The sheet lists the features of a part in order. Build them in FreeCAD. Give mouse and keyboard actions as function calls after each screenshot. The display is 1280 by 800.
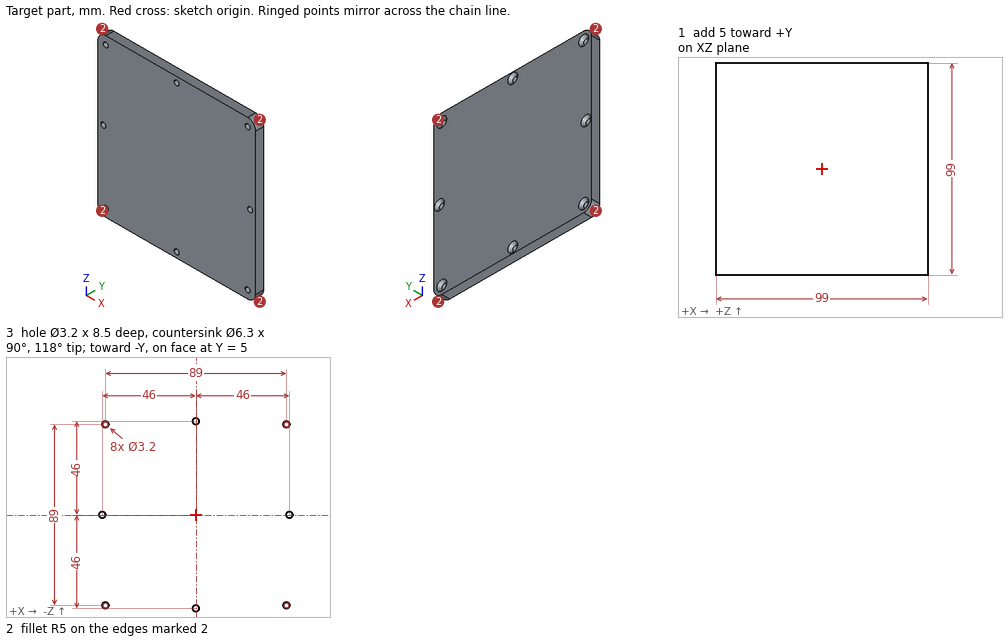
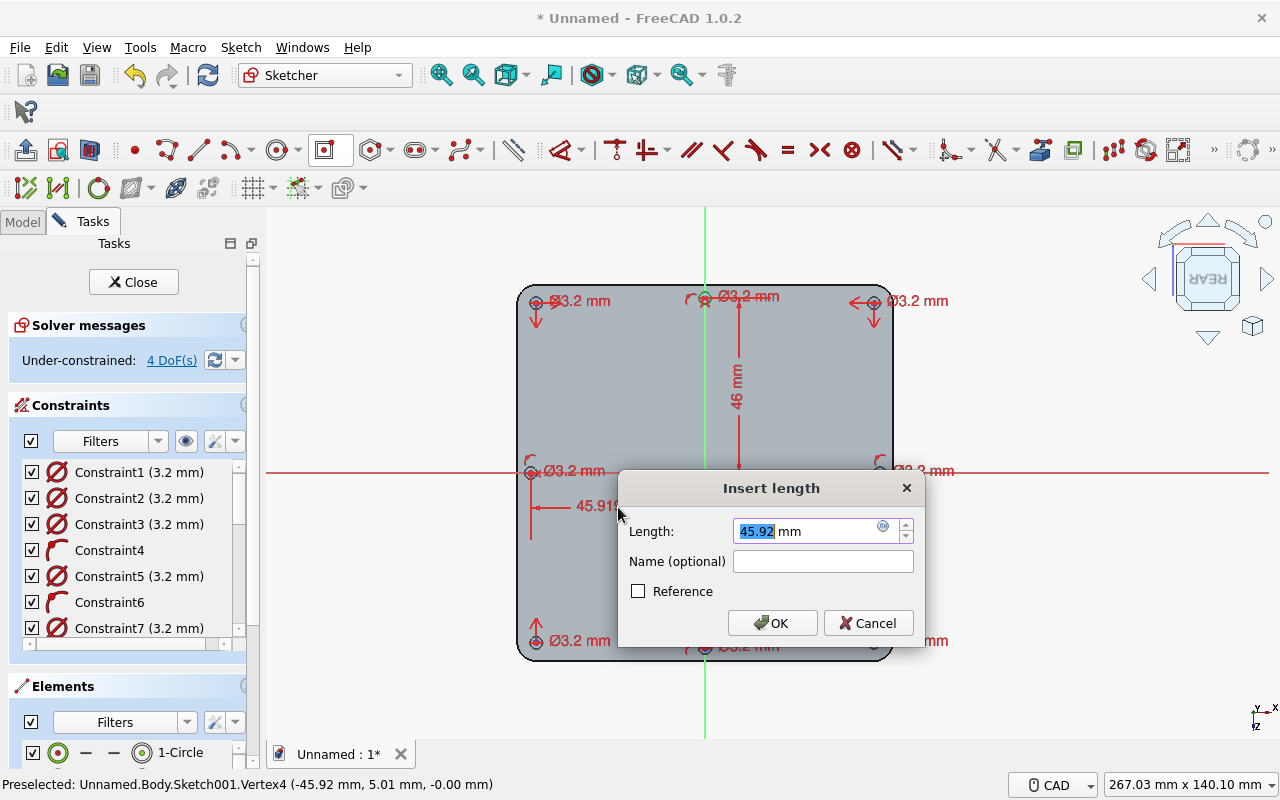
text(46)
key(Return)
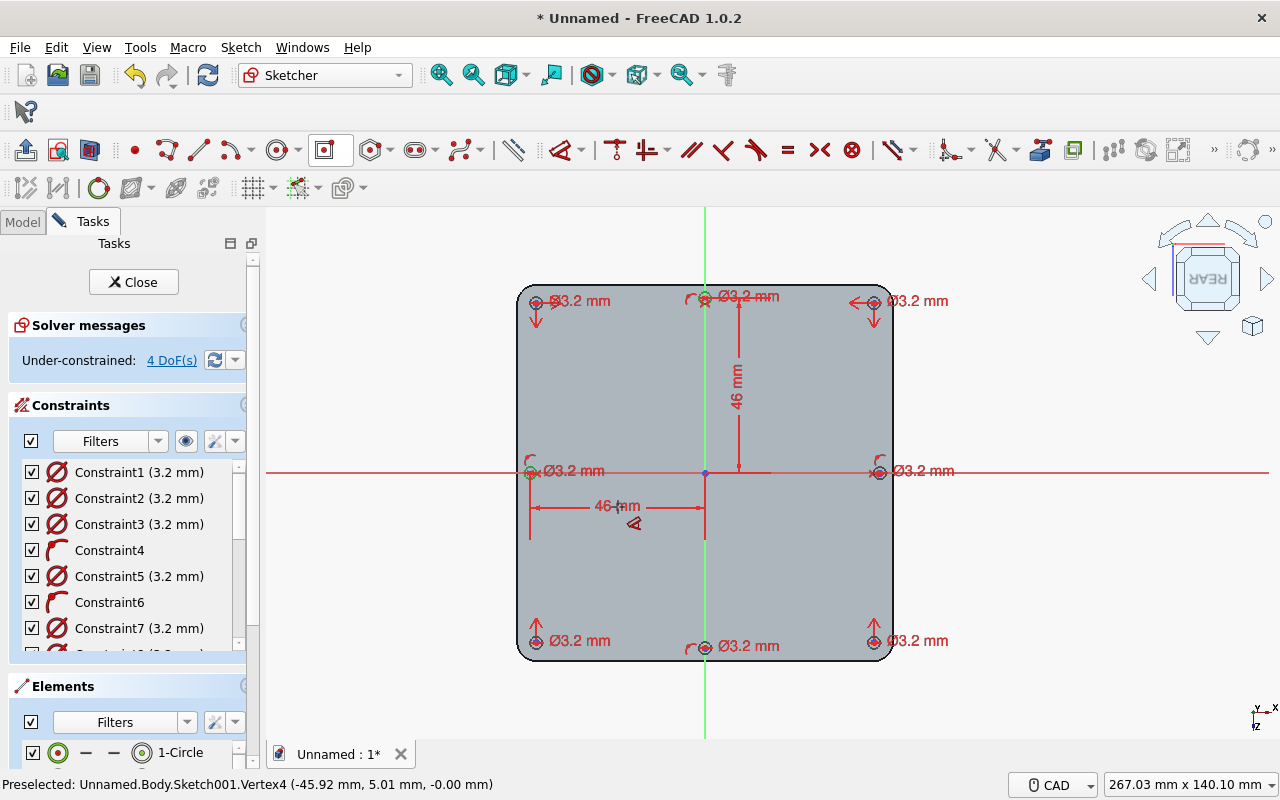
click(705, 648)
click(739, 561)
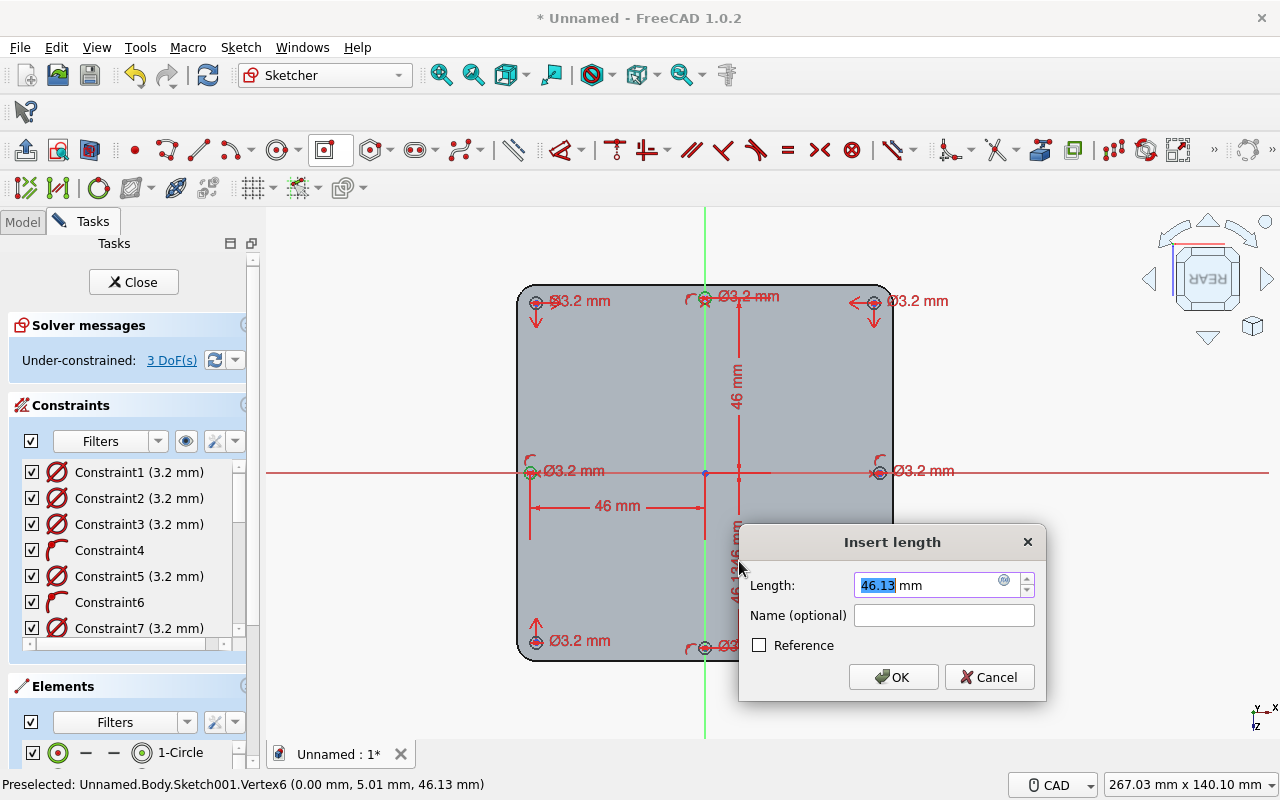
text(46)
key(Return)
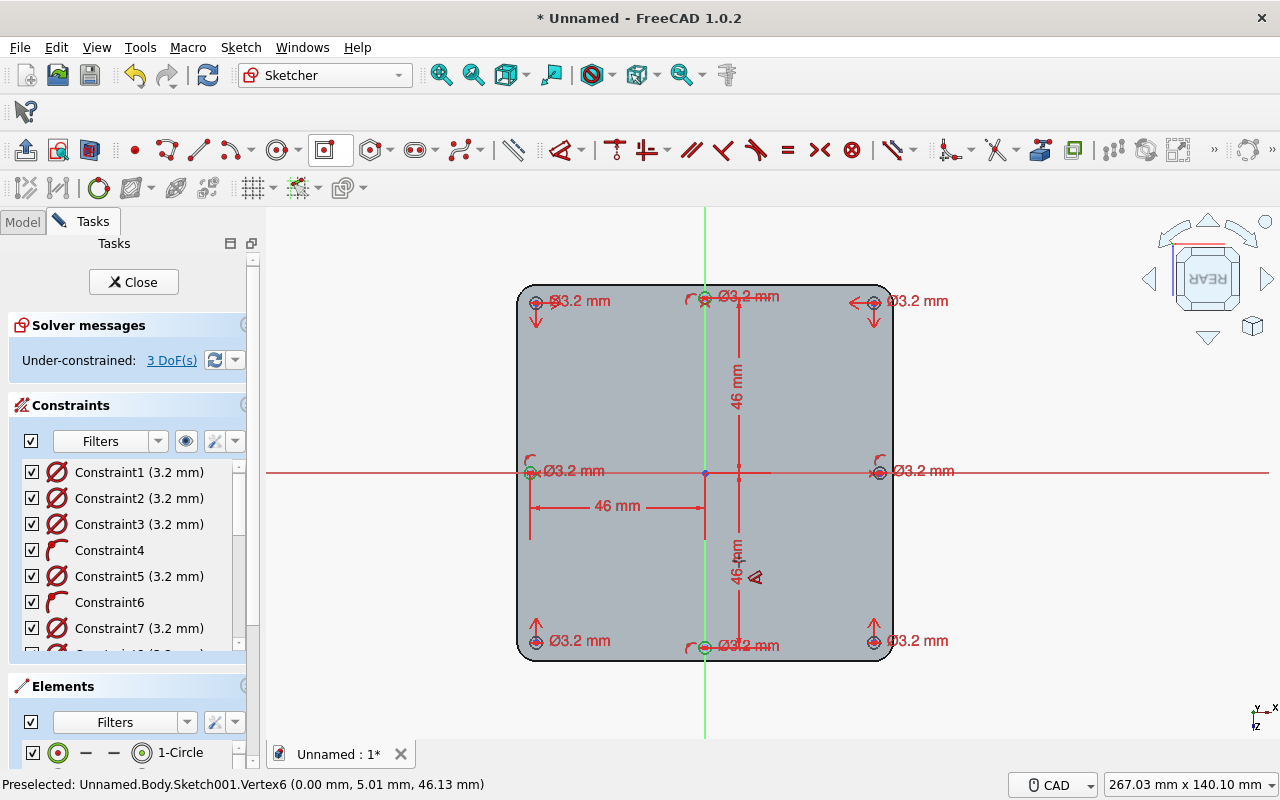
click(880, 473)
click(793, 507)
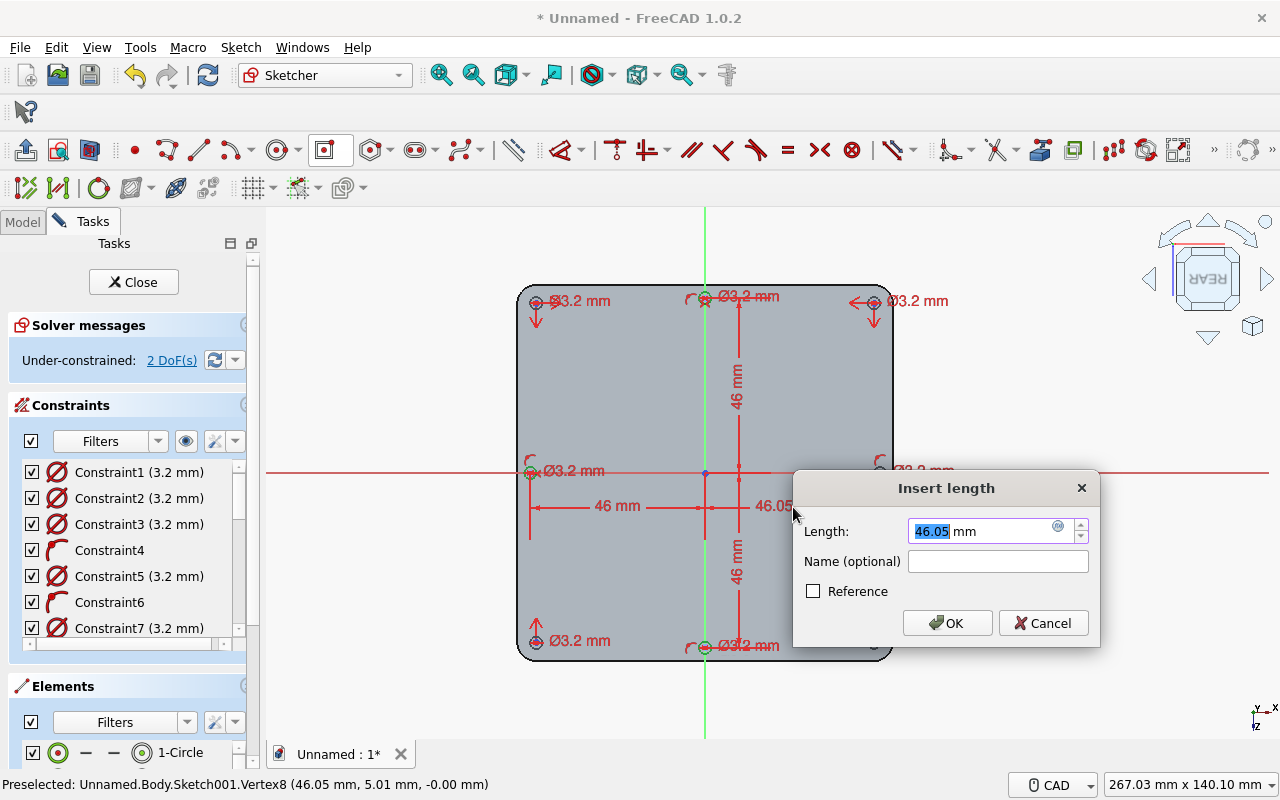
text(46)
key(Return)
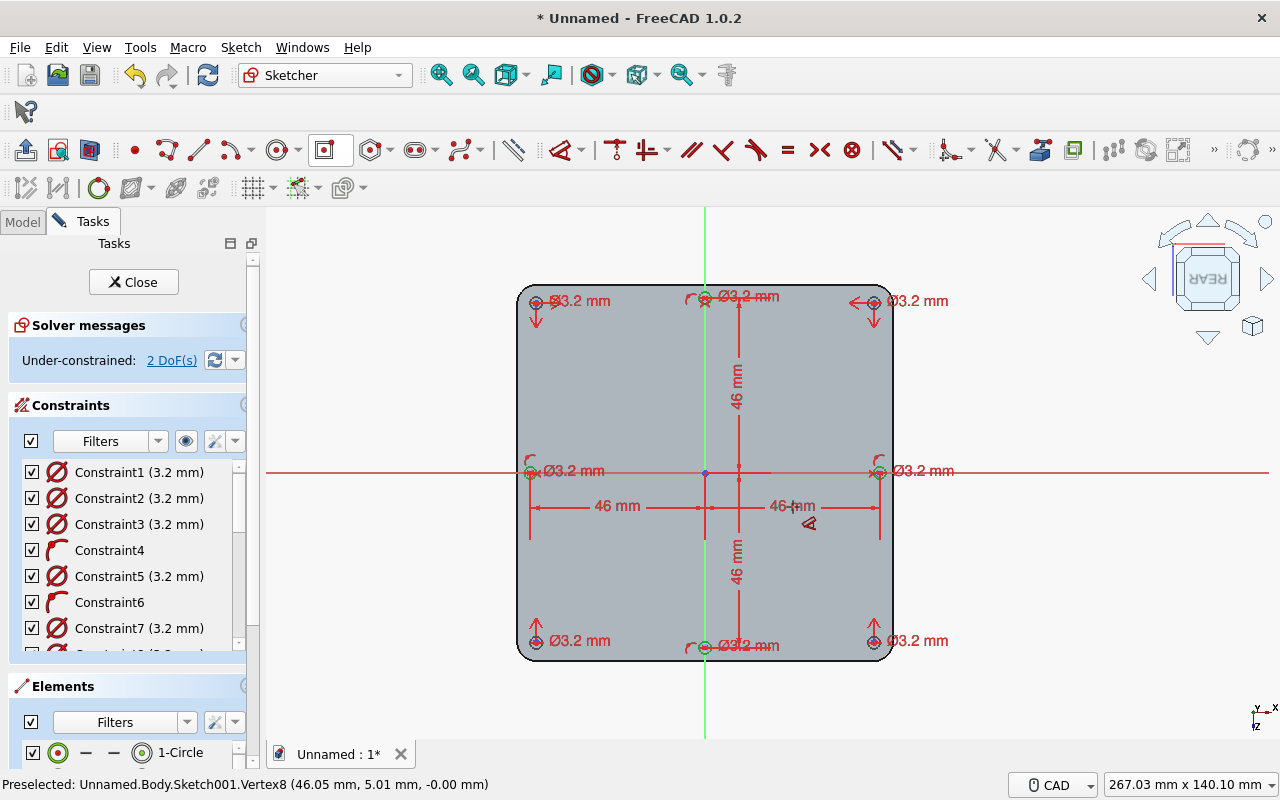
click(536, 303)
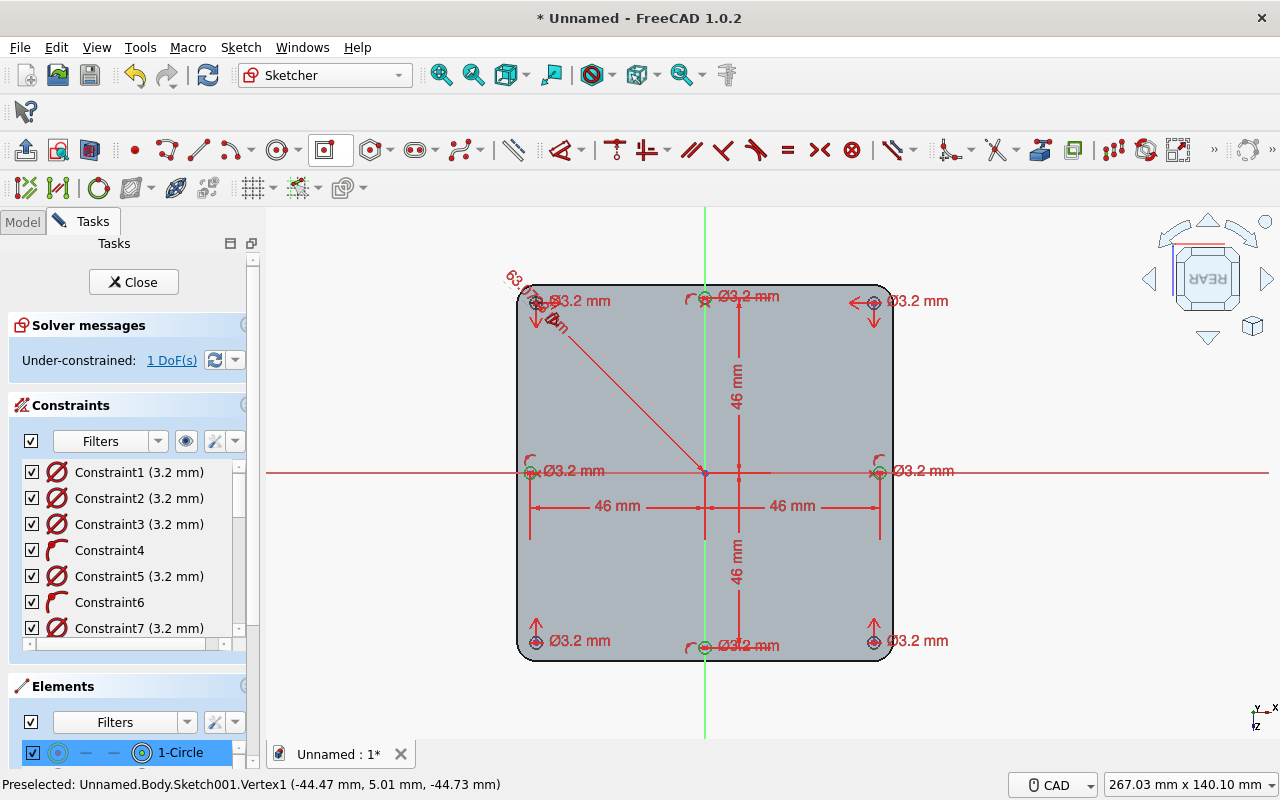
click(874, 303)
click(627, 269)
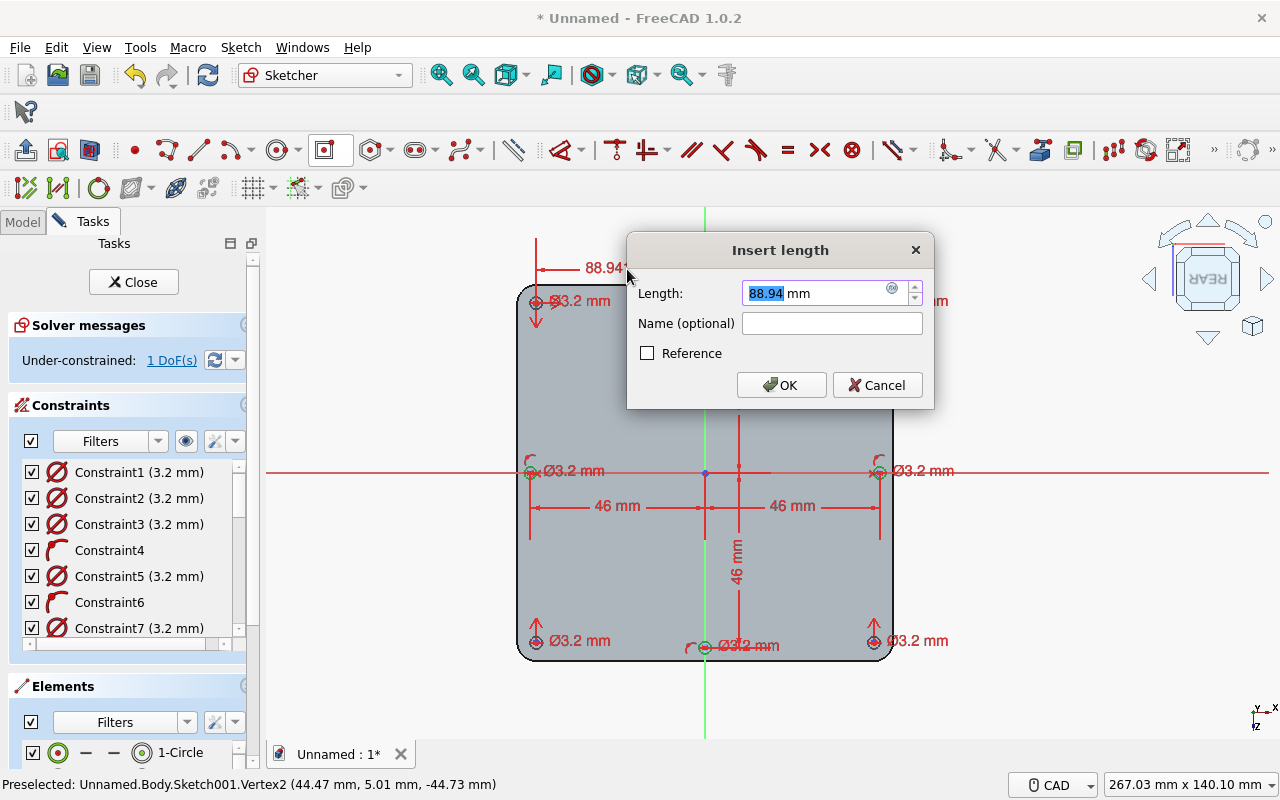
text(89)
key(Return)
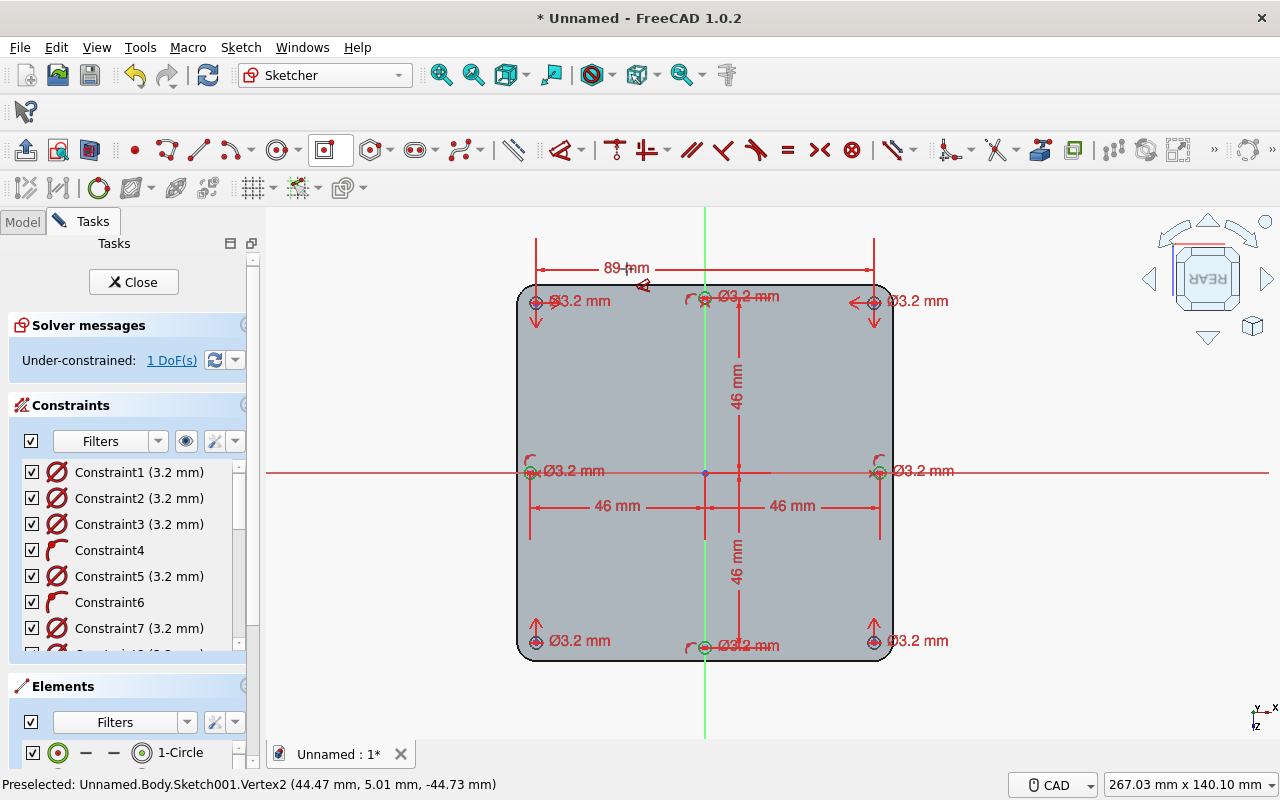
click(536, 303)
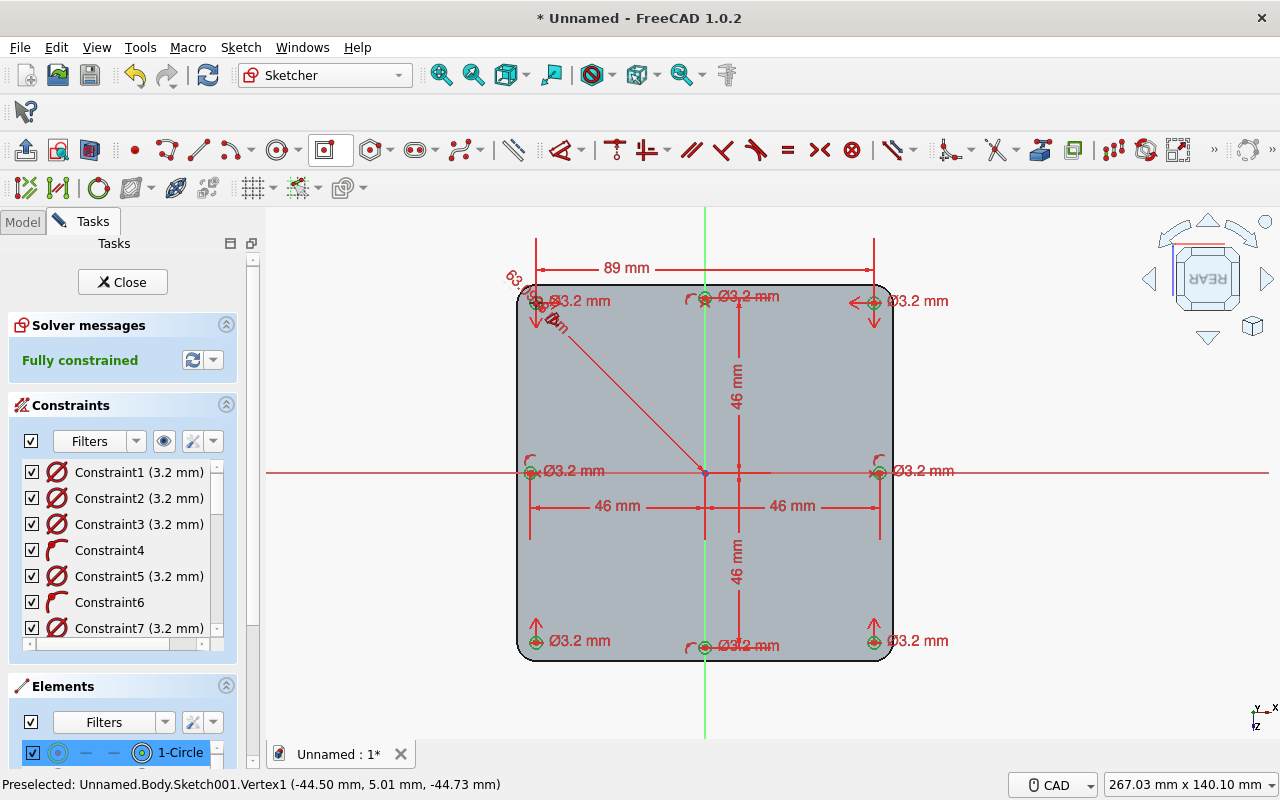
click(536, 643)
click(502, 395)